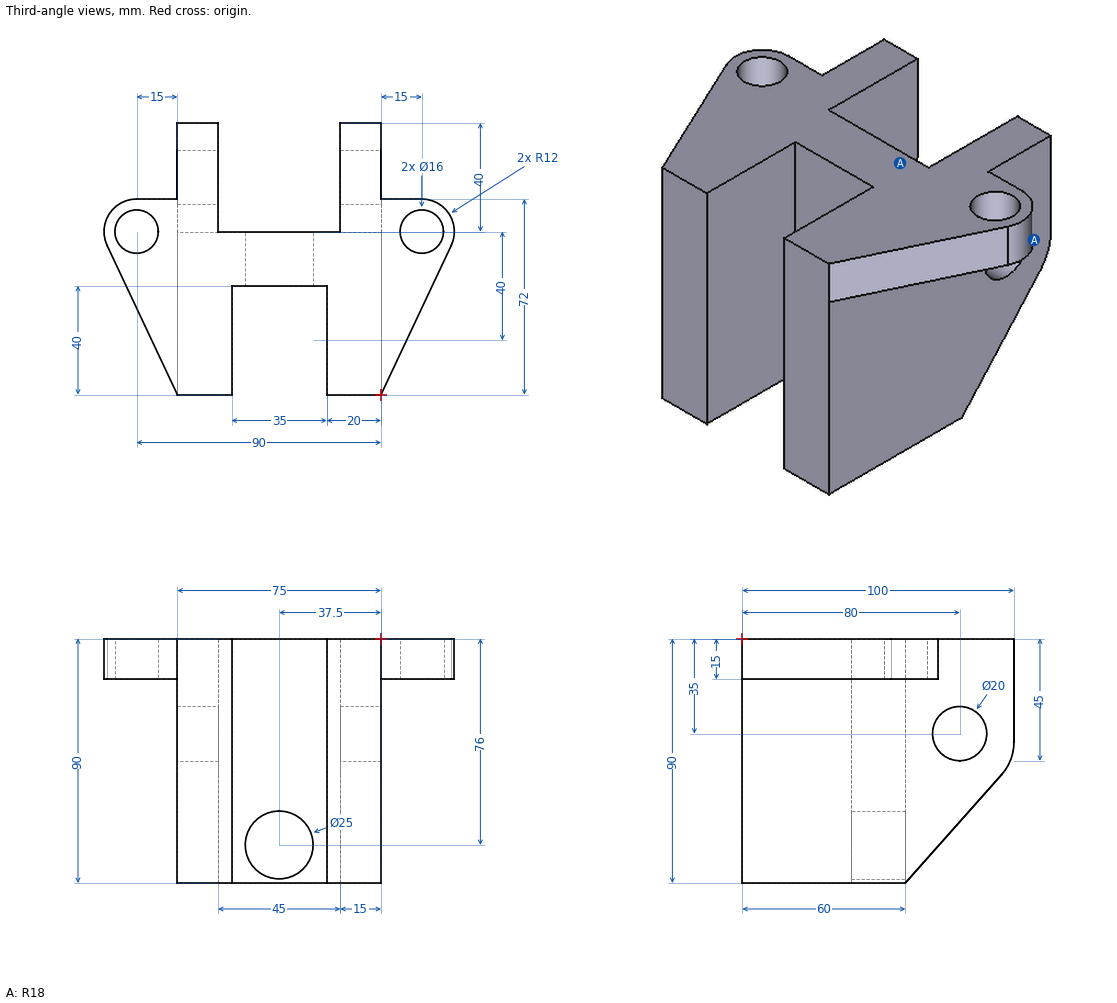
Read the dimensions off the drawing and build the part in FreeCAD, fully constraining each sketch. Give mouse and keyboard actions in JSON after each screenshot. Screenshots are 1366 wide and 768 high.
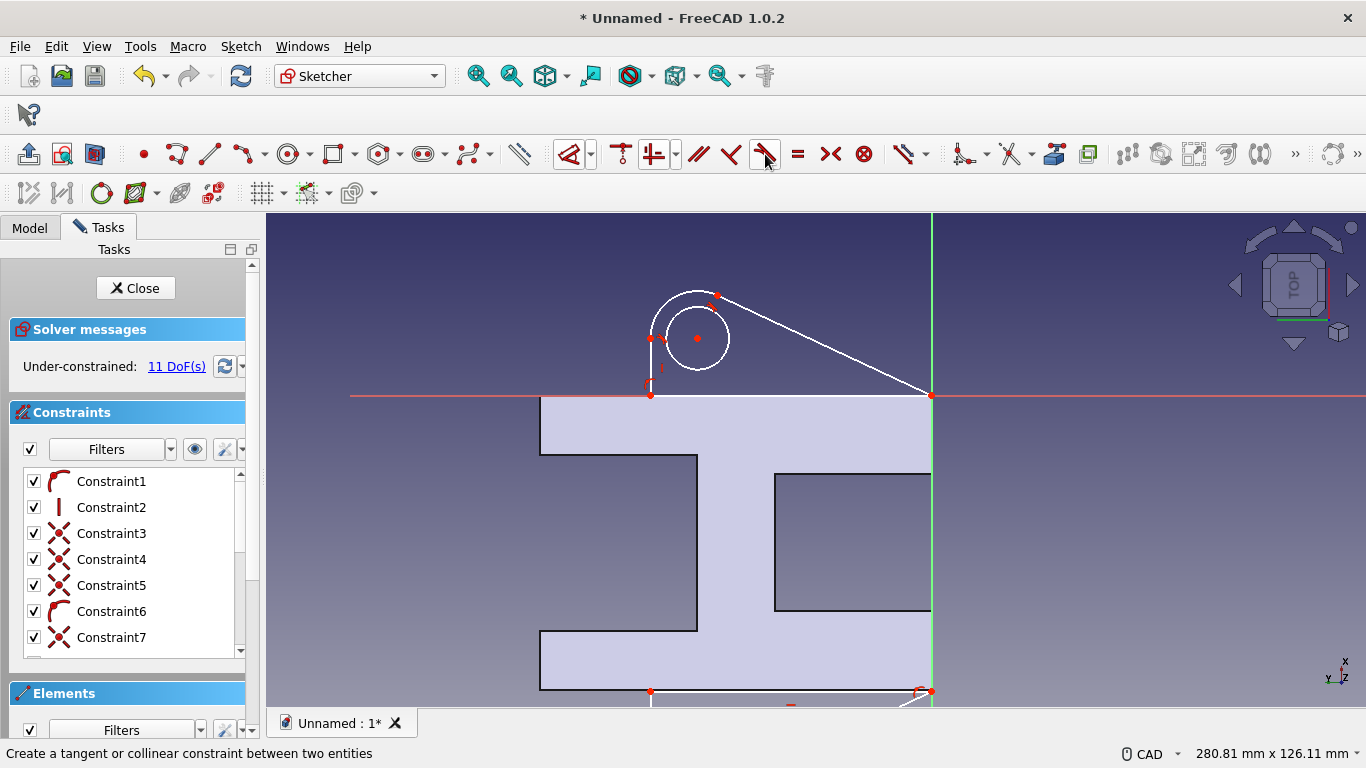
{"action": "scroll", "coordinate": [659, 292], "scroll_direction": "down", "scroll_amount": 2}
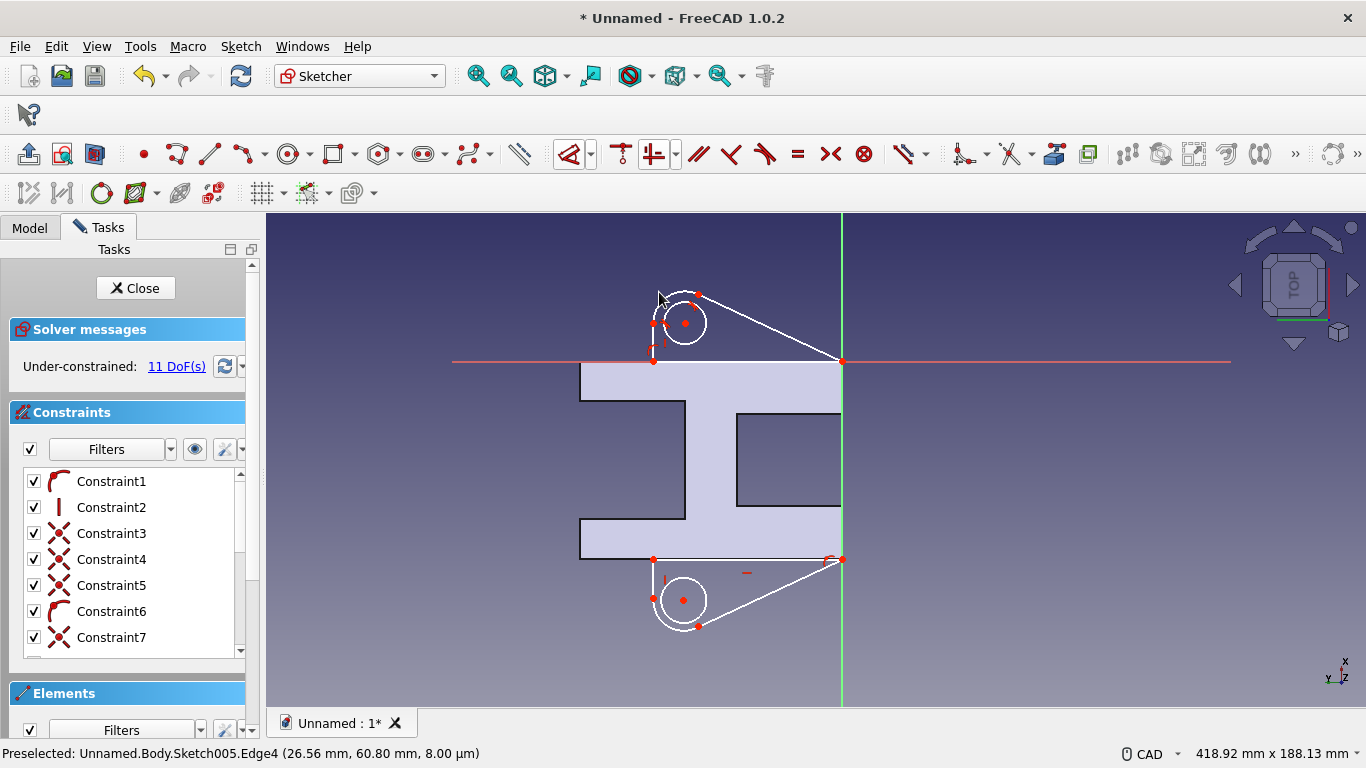
{"action": "left_click", "coordinate": [742, 607]}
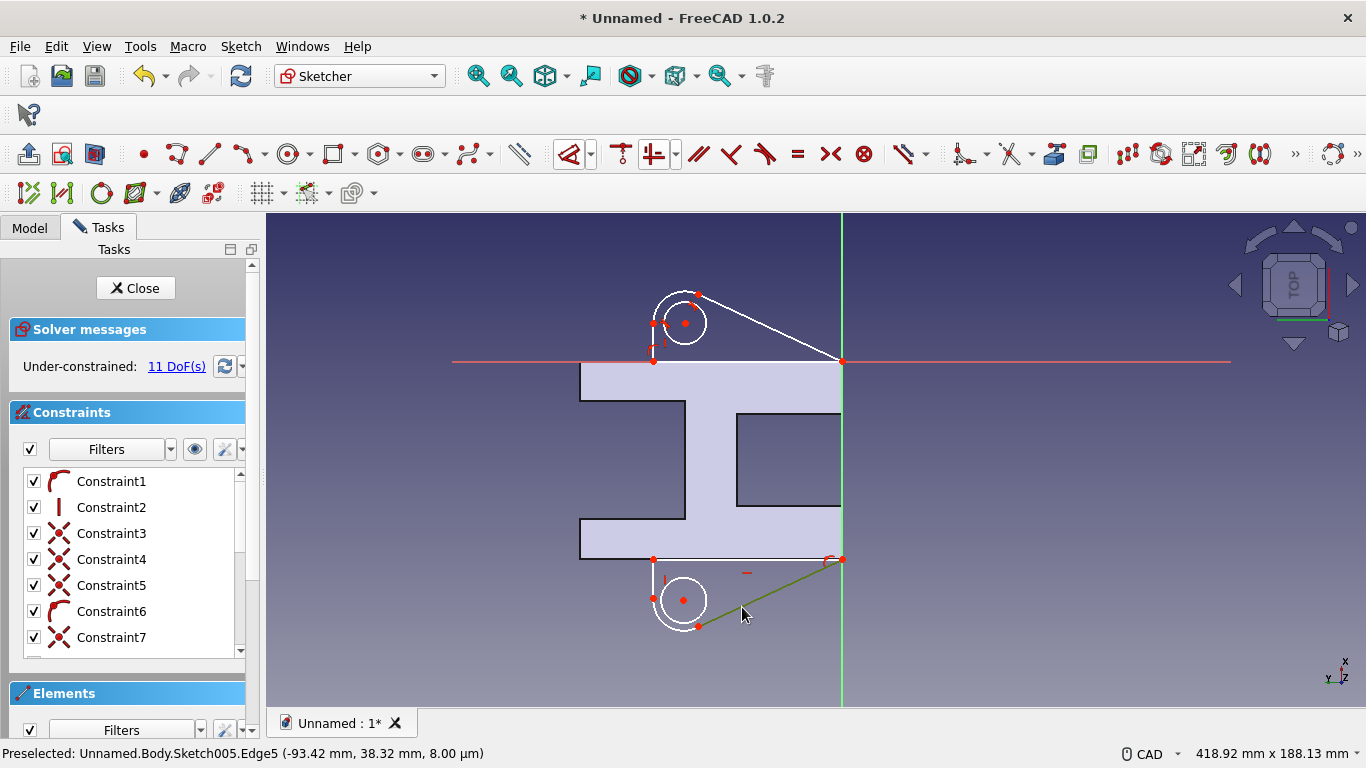
{"action": "scroll", "coordinate": [680, 631], "scroll_direction": "up", "scroll_amount": 3}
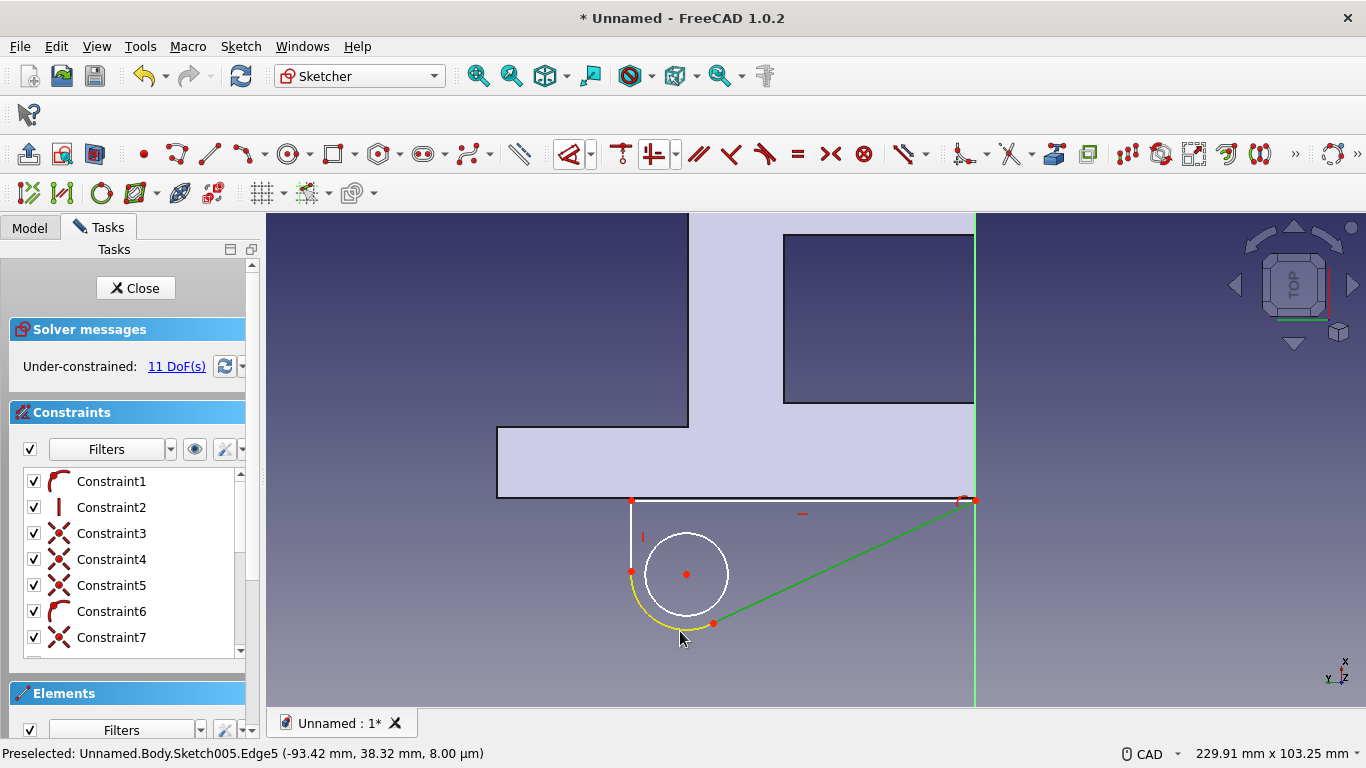
{"action": "left_click", "coordinate": [679, 629]}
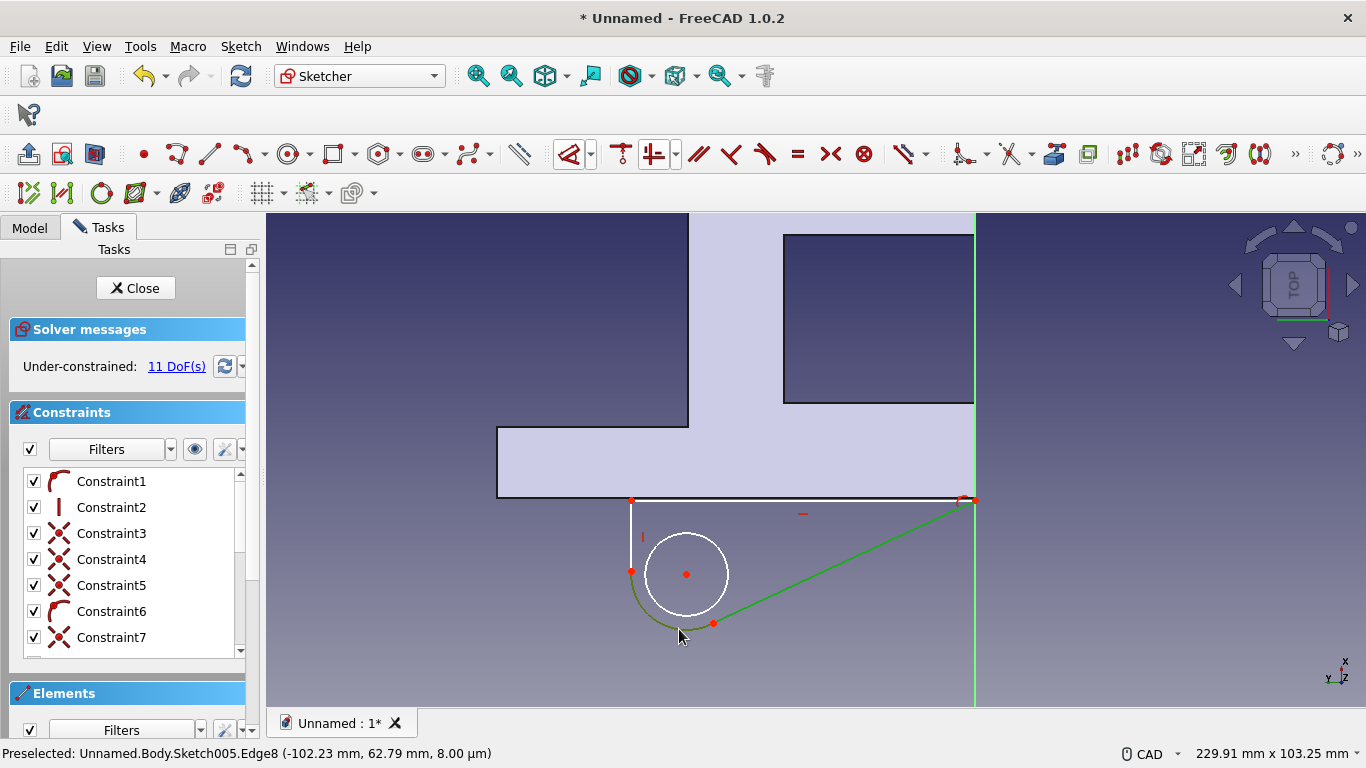
{"action": "left_click", "coordinate": [765, 154]}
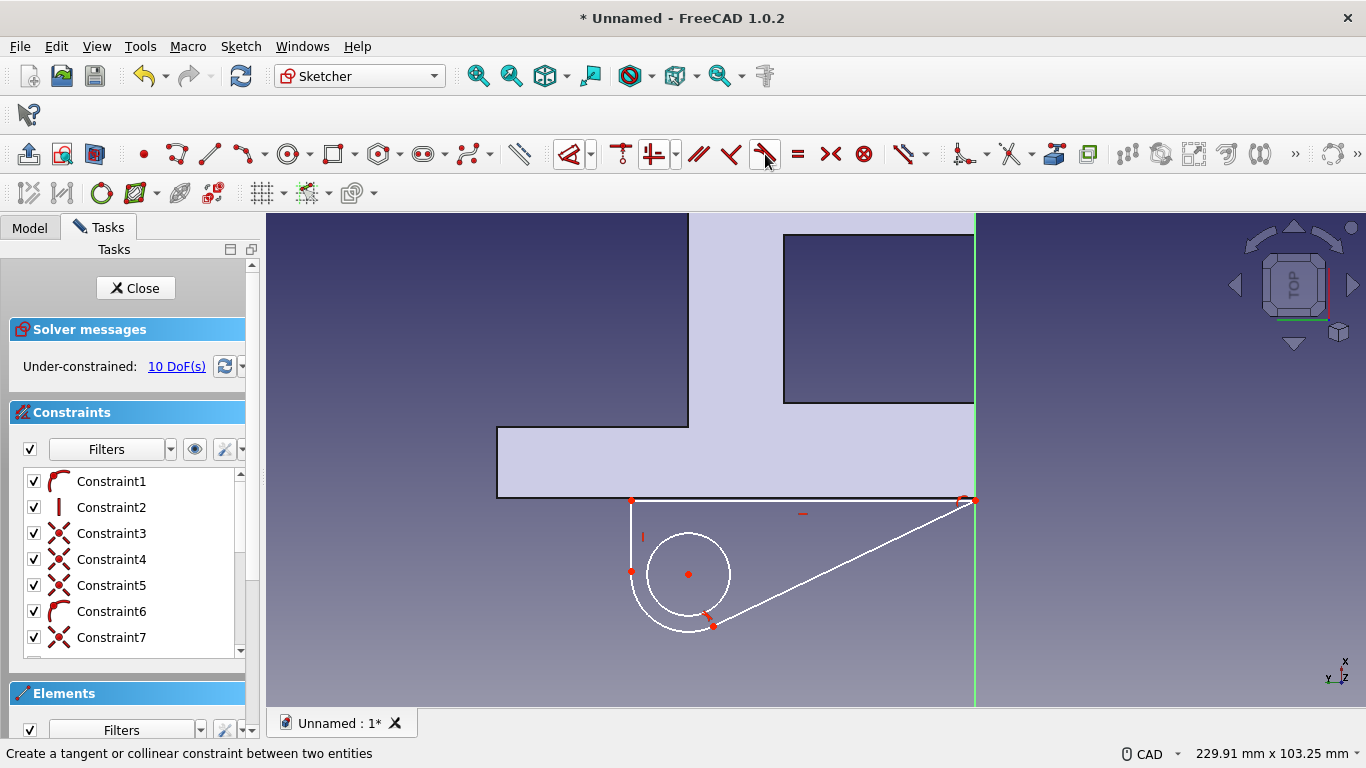
{"action": "left_click", "coordinate": [631, 522]}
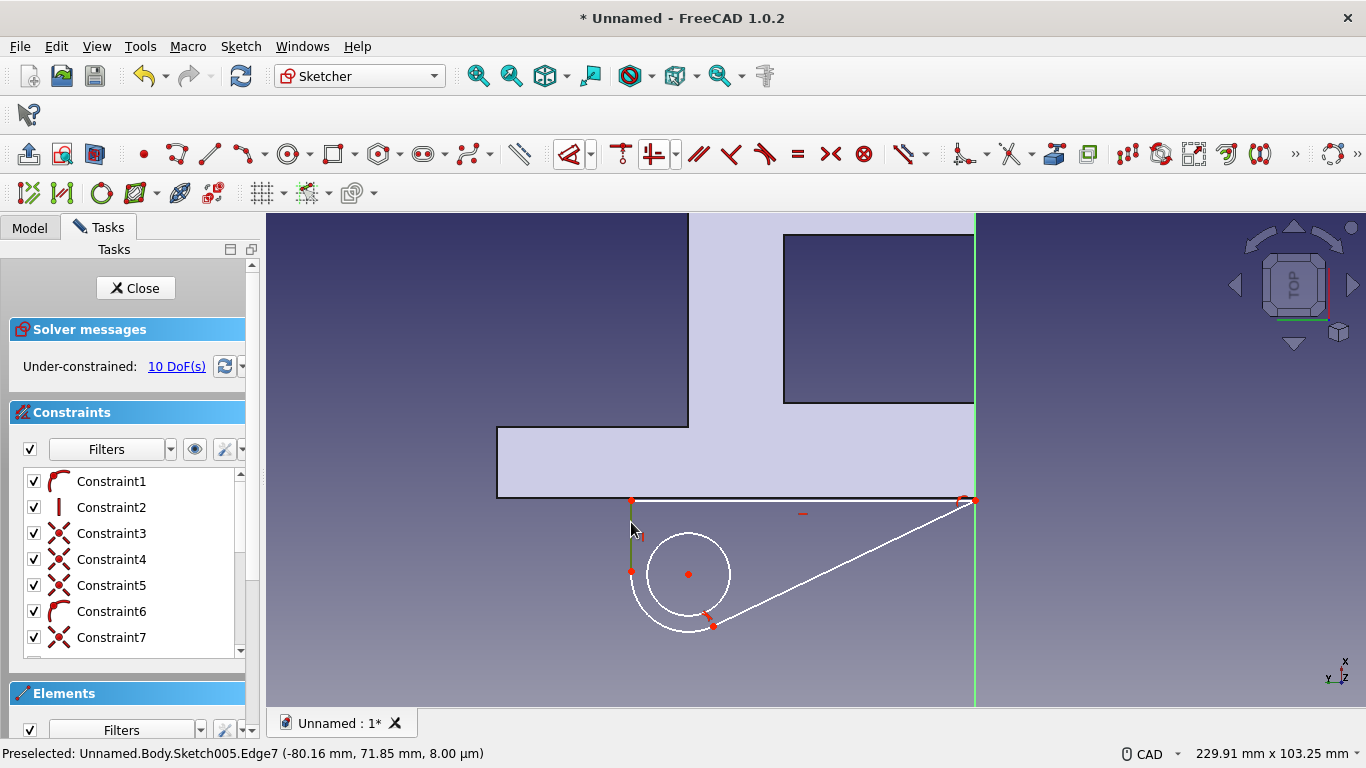
{"action": "left_click", "coordinate": [640, 606]}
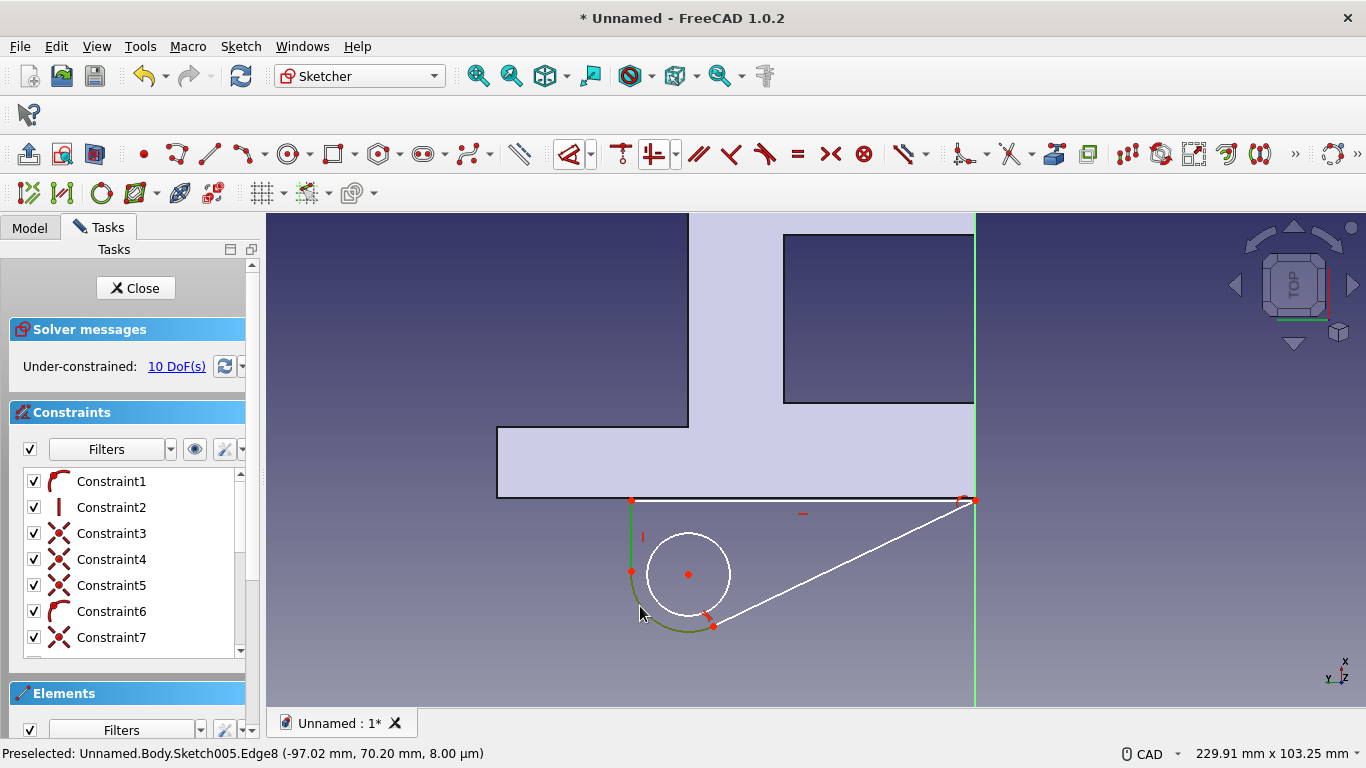
{"action": "left_click", "coordinate": [765, 154]}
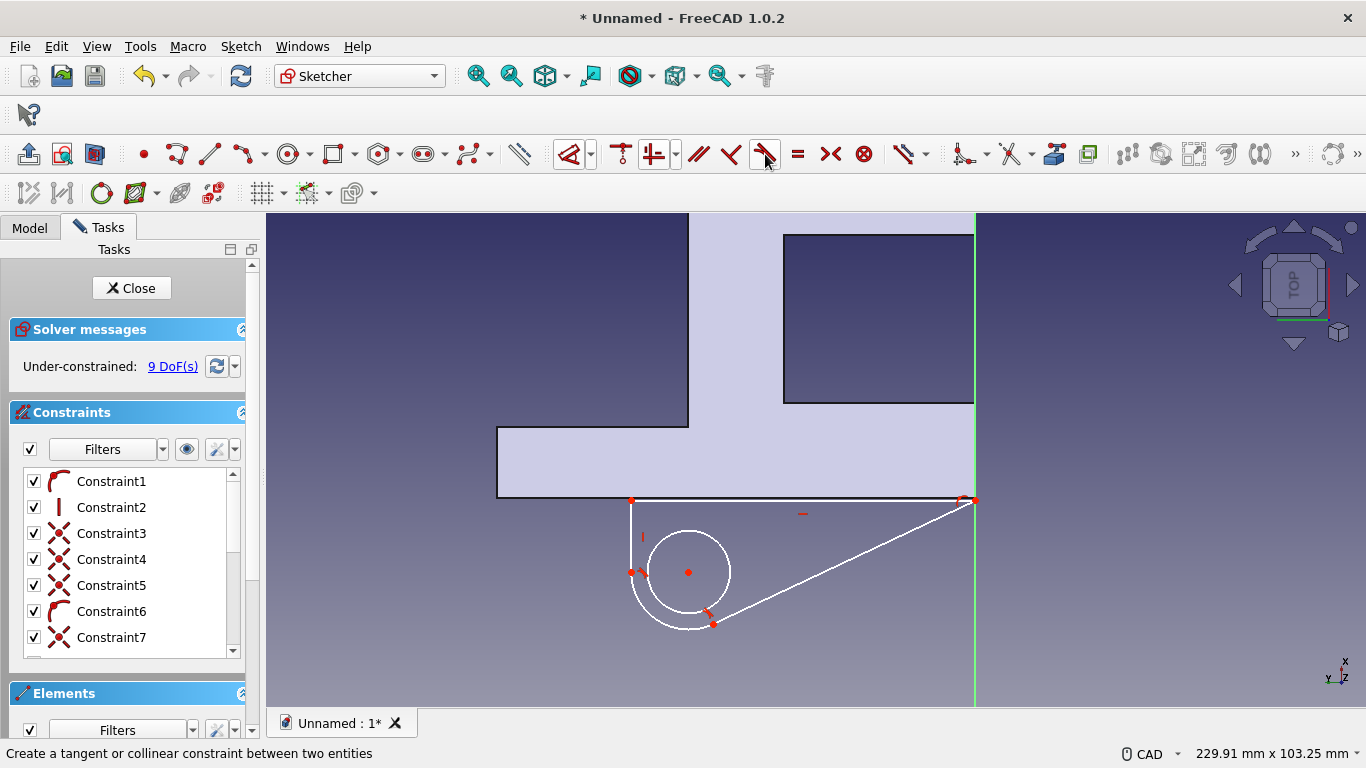
{"action": "scroll", "coordinate": [680, 632], "scroll_direction": "down", "scroll_amount": 3}